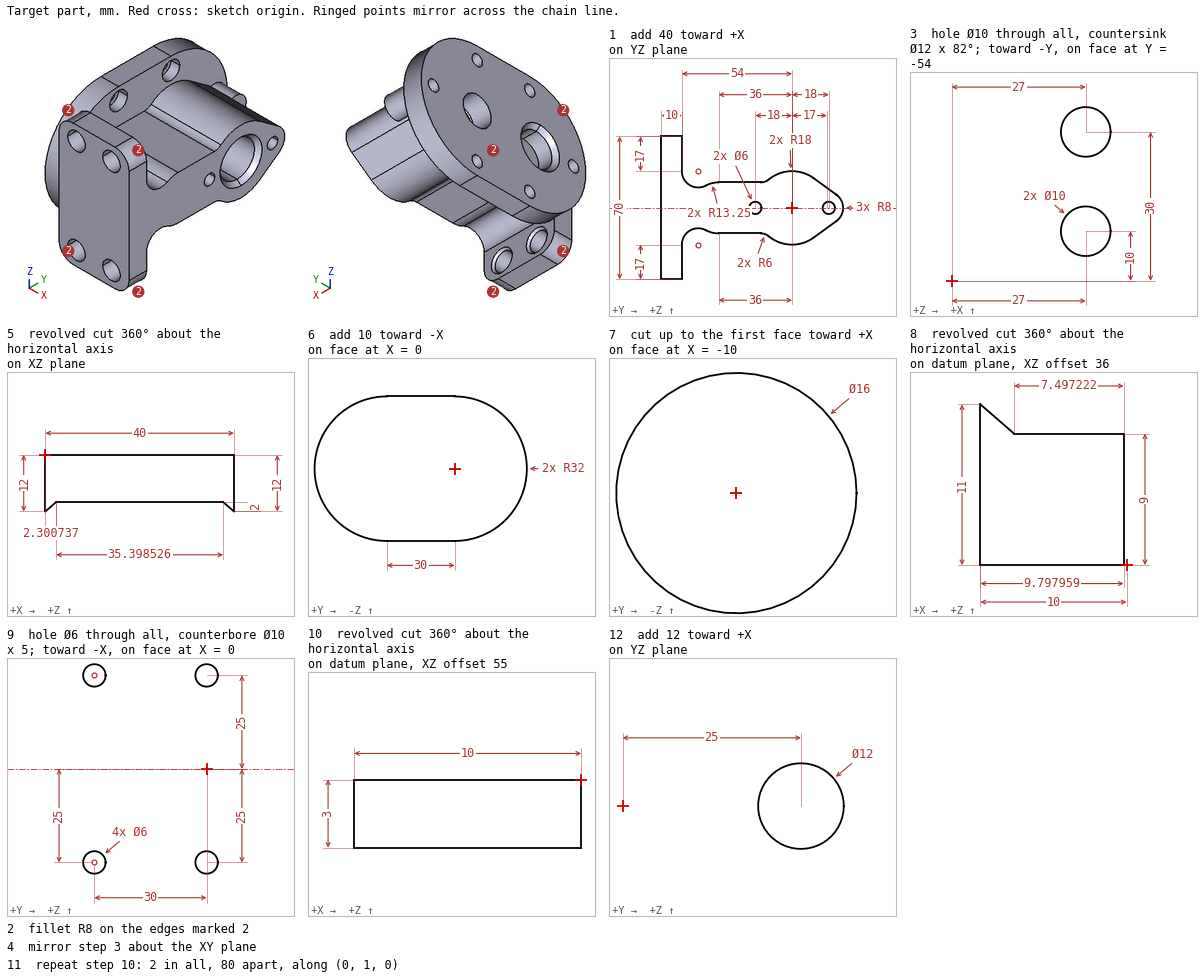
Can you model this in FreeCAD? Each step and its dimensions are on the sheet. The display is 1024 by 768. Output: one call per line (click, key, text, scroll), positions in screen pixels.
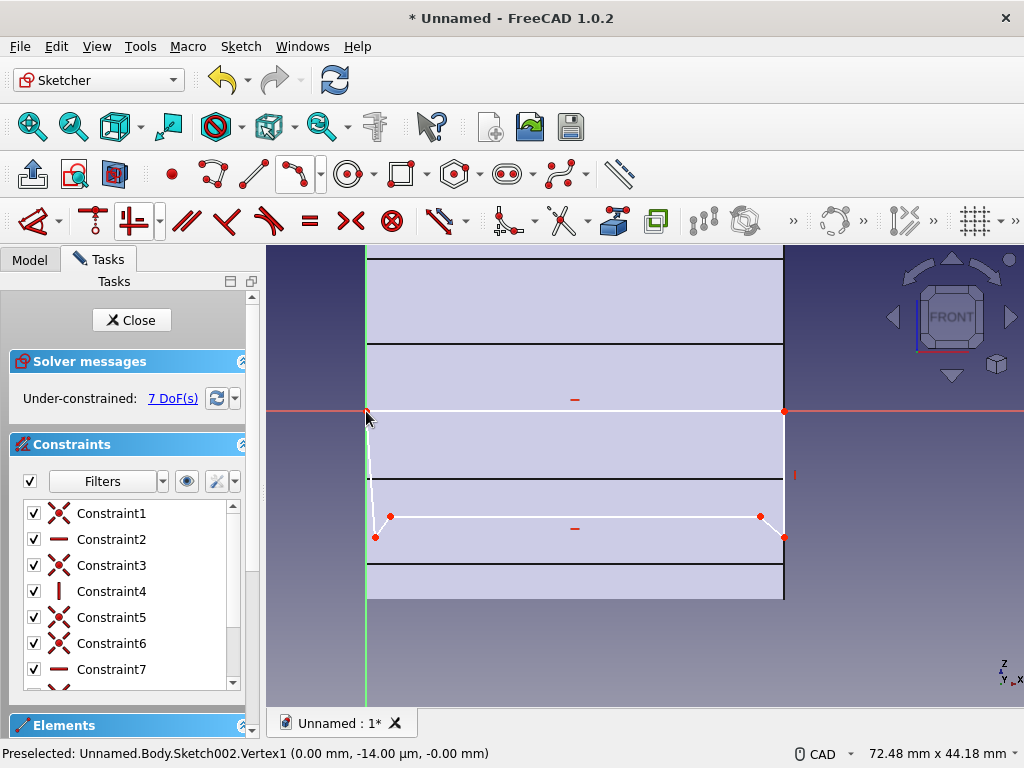
click(369, 449)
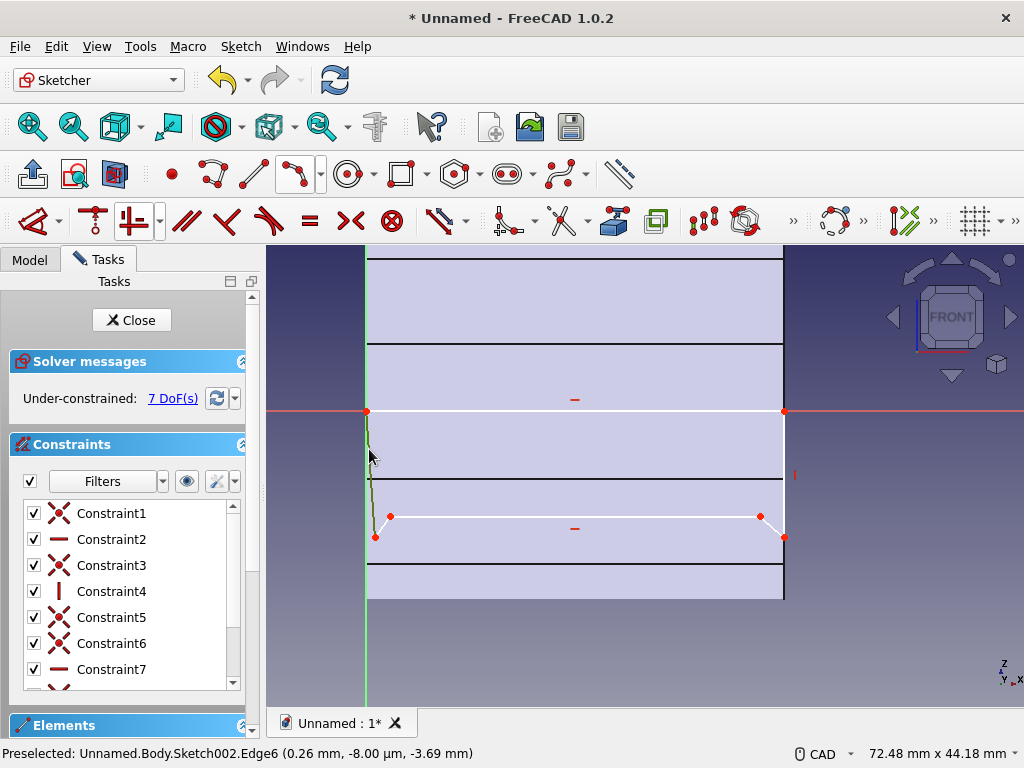
click(160, 222)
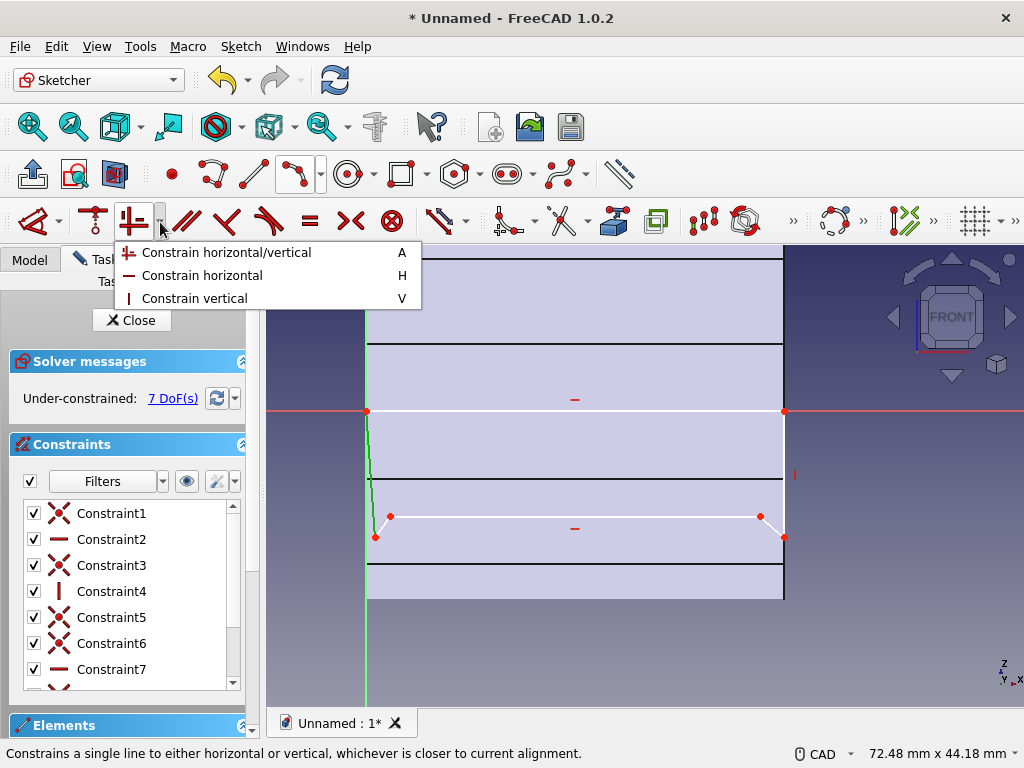
click(268, 298)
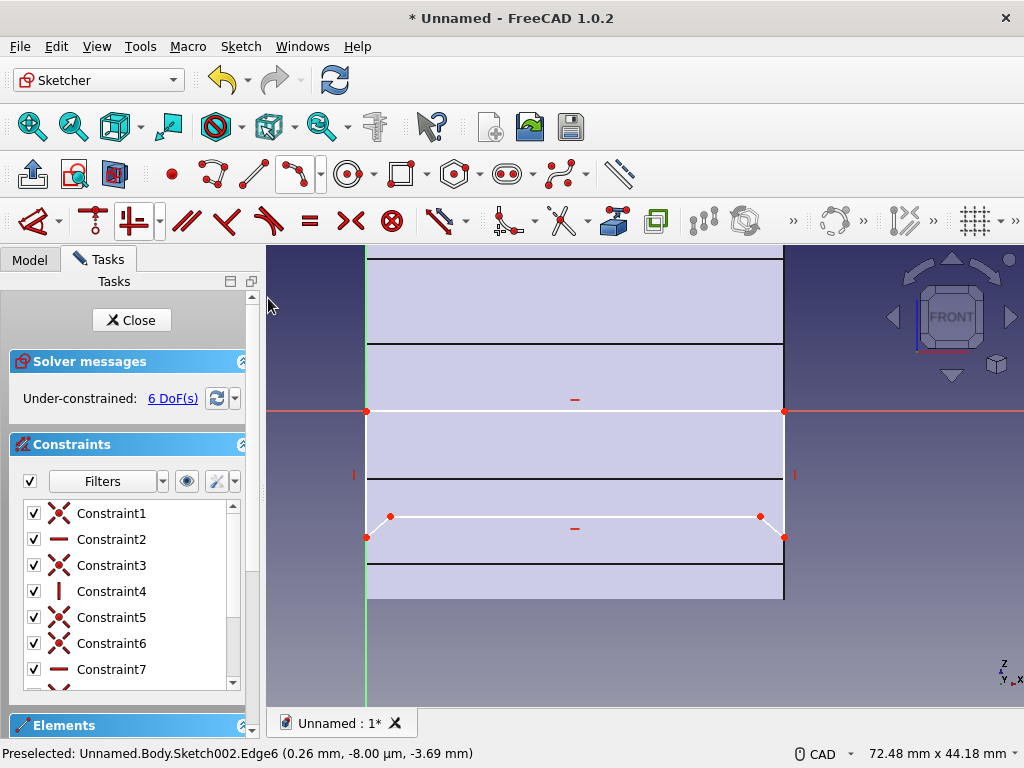
click(32, 222)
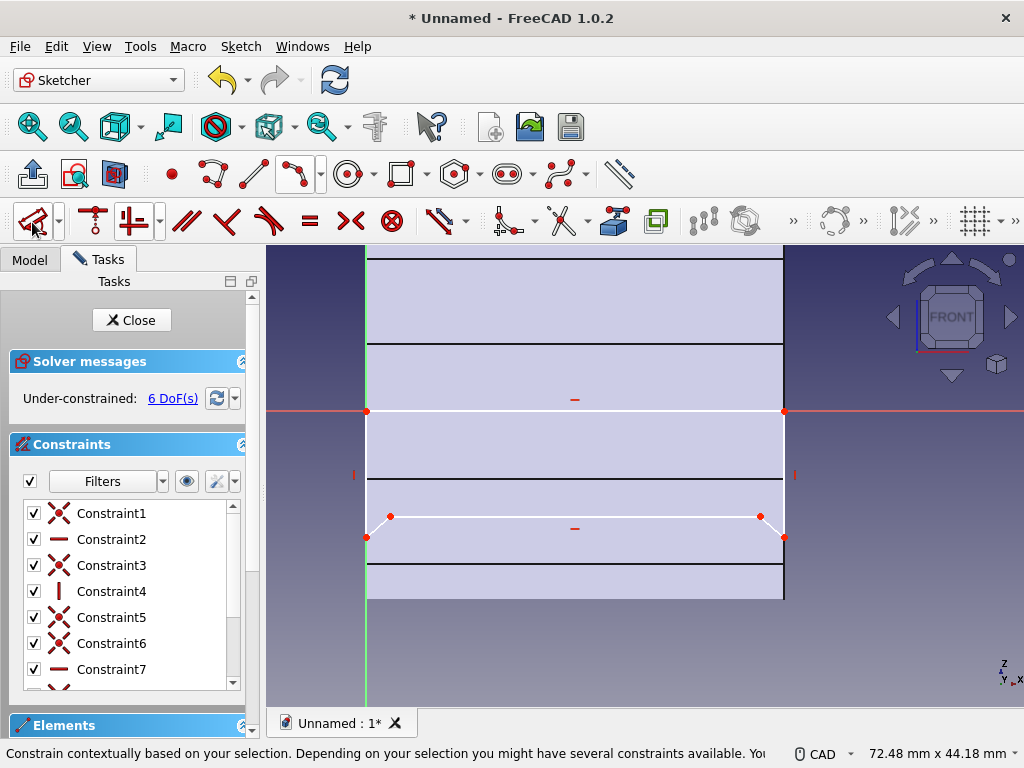
click(492, 411)
click(575, 377)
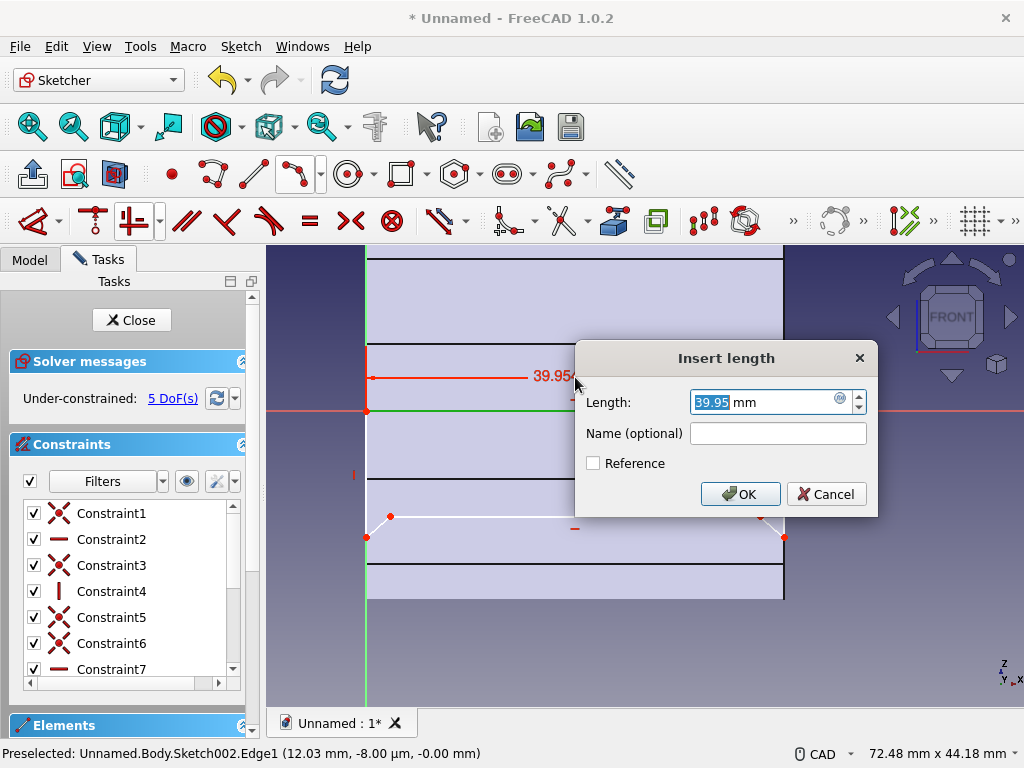
text(40)
key(Return)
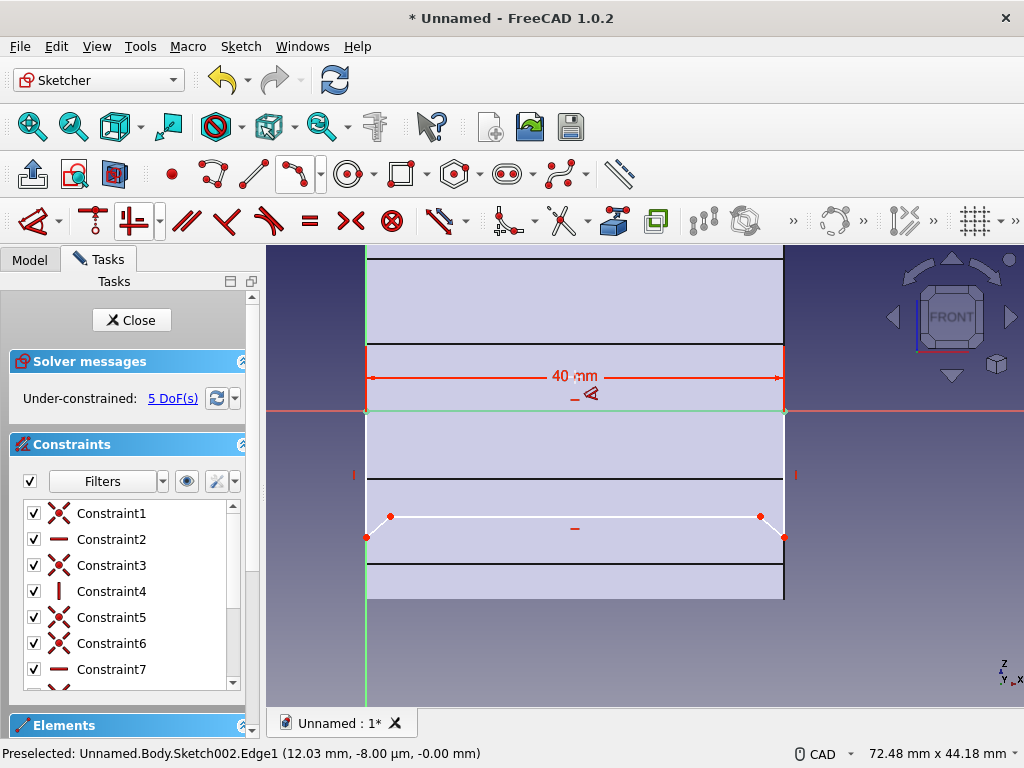
click(784, 449)
click(818, 475)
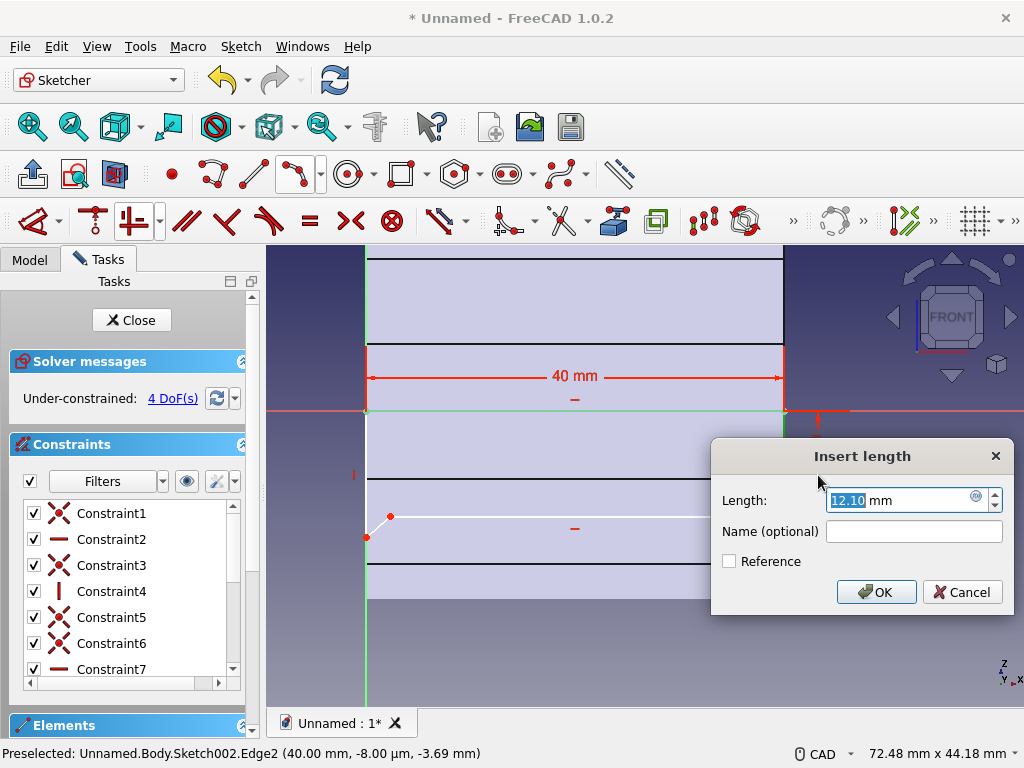
text(12)
key(Return)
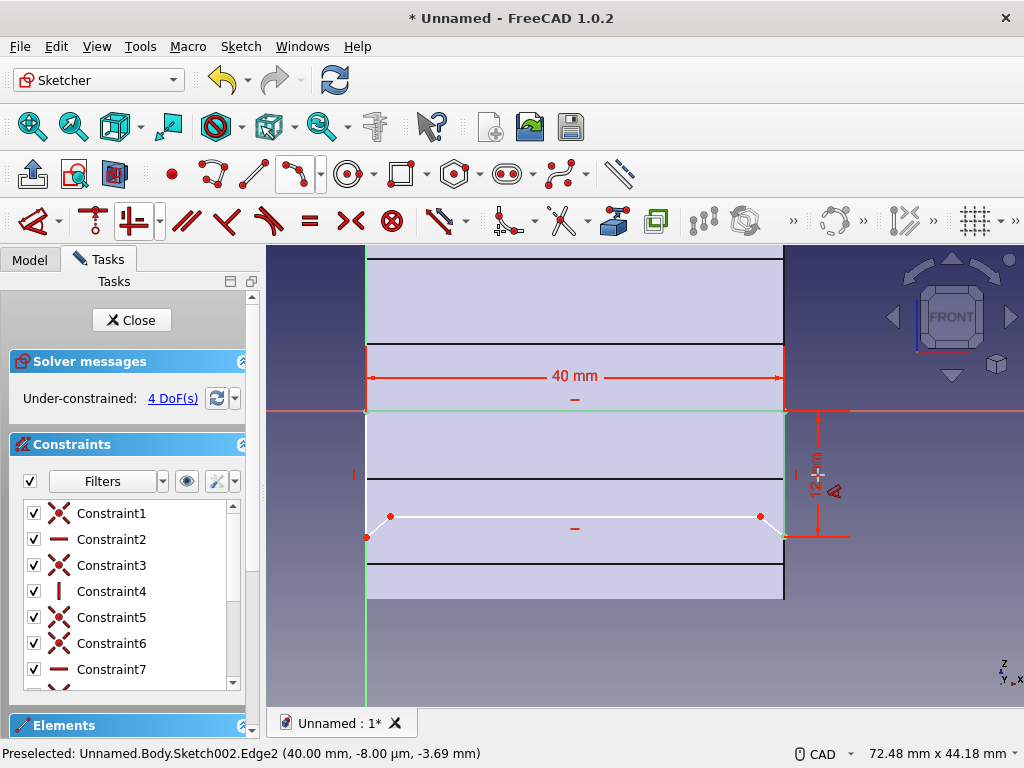
click(366, 500)
click(332, 475)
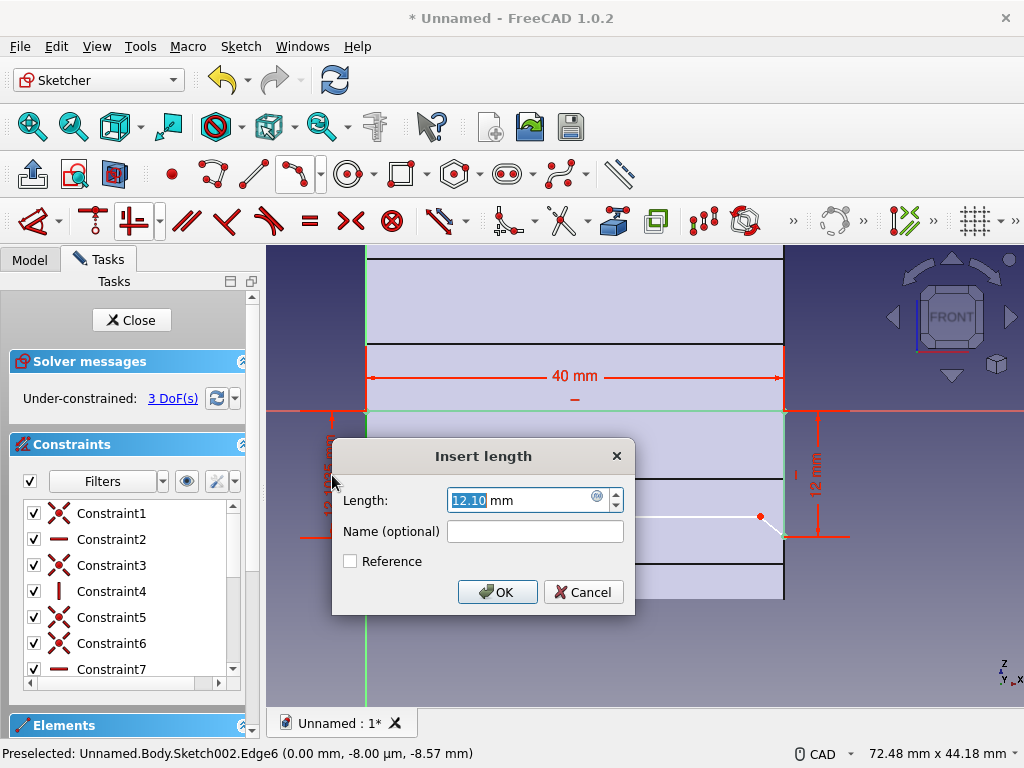
text(12)
key(Return)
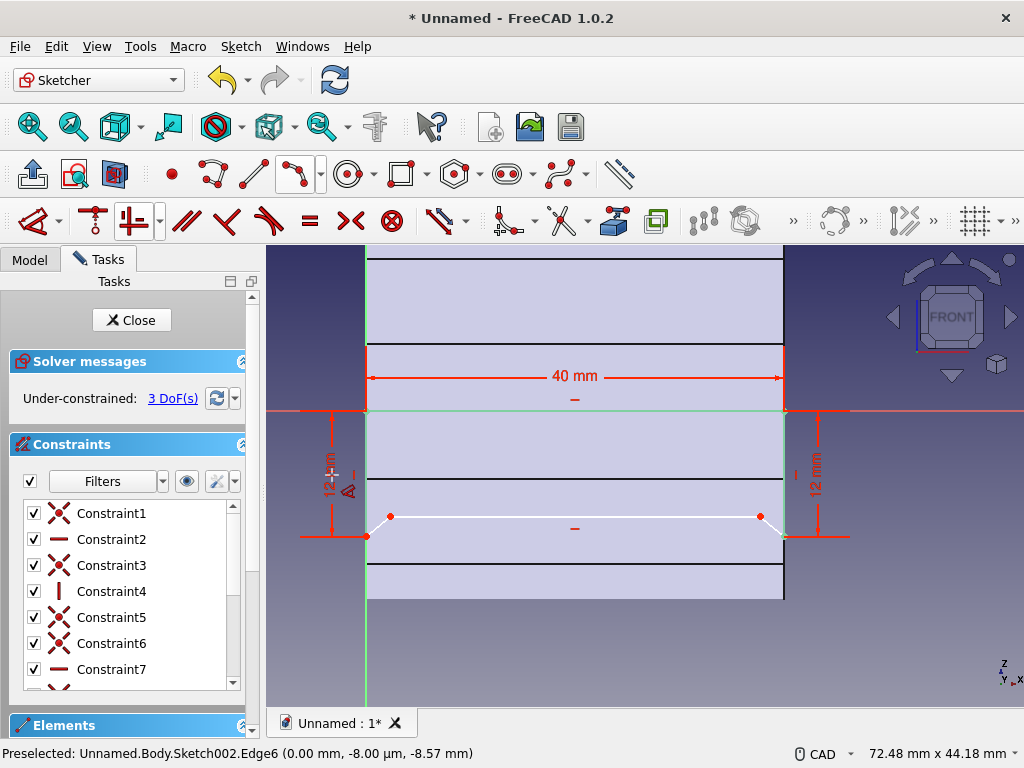
scroll(767, 523, up, 4)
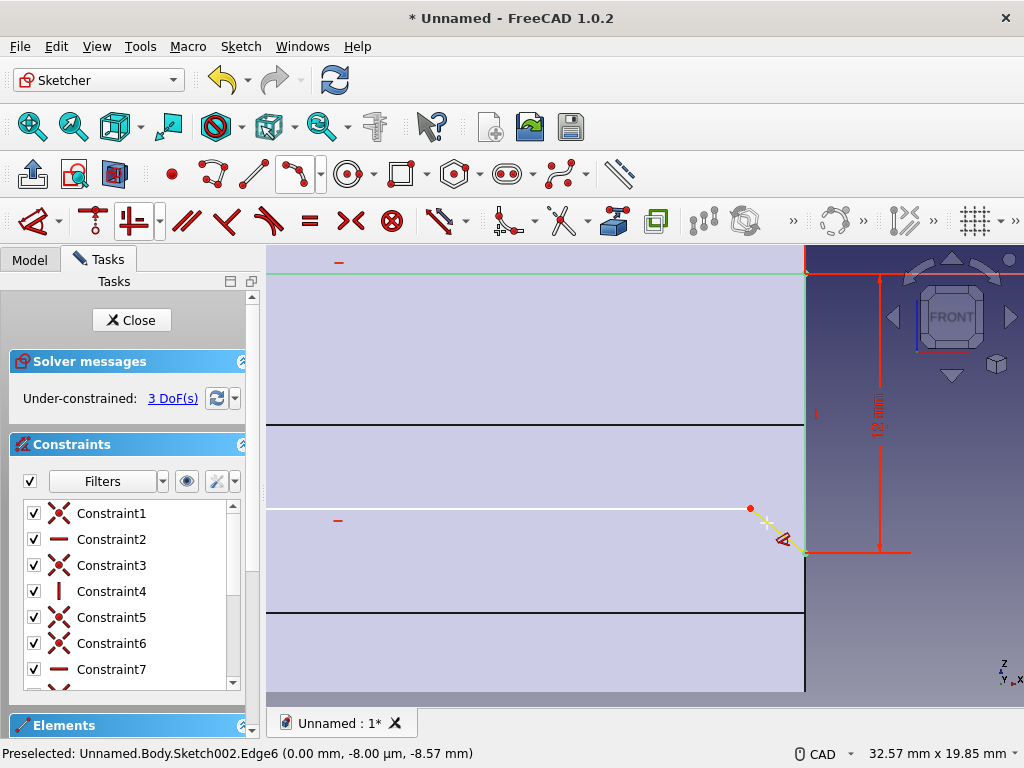
click(767, 522)
click(839, 531)